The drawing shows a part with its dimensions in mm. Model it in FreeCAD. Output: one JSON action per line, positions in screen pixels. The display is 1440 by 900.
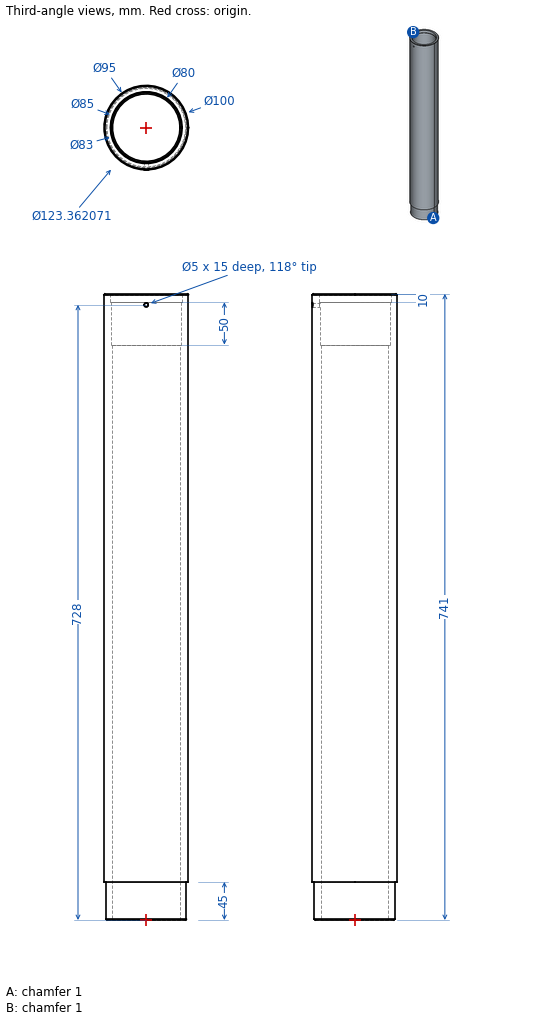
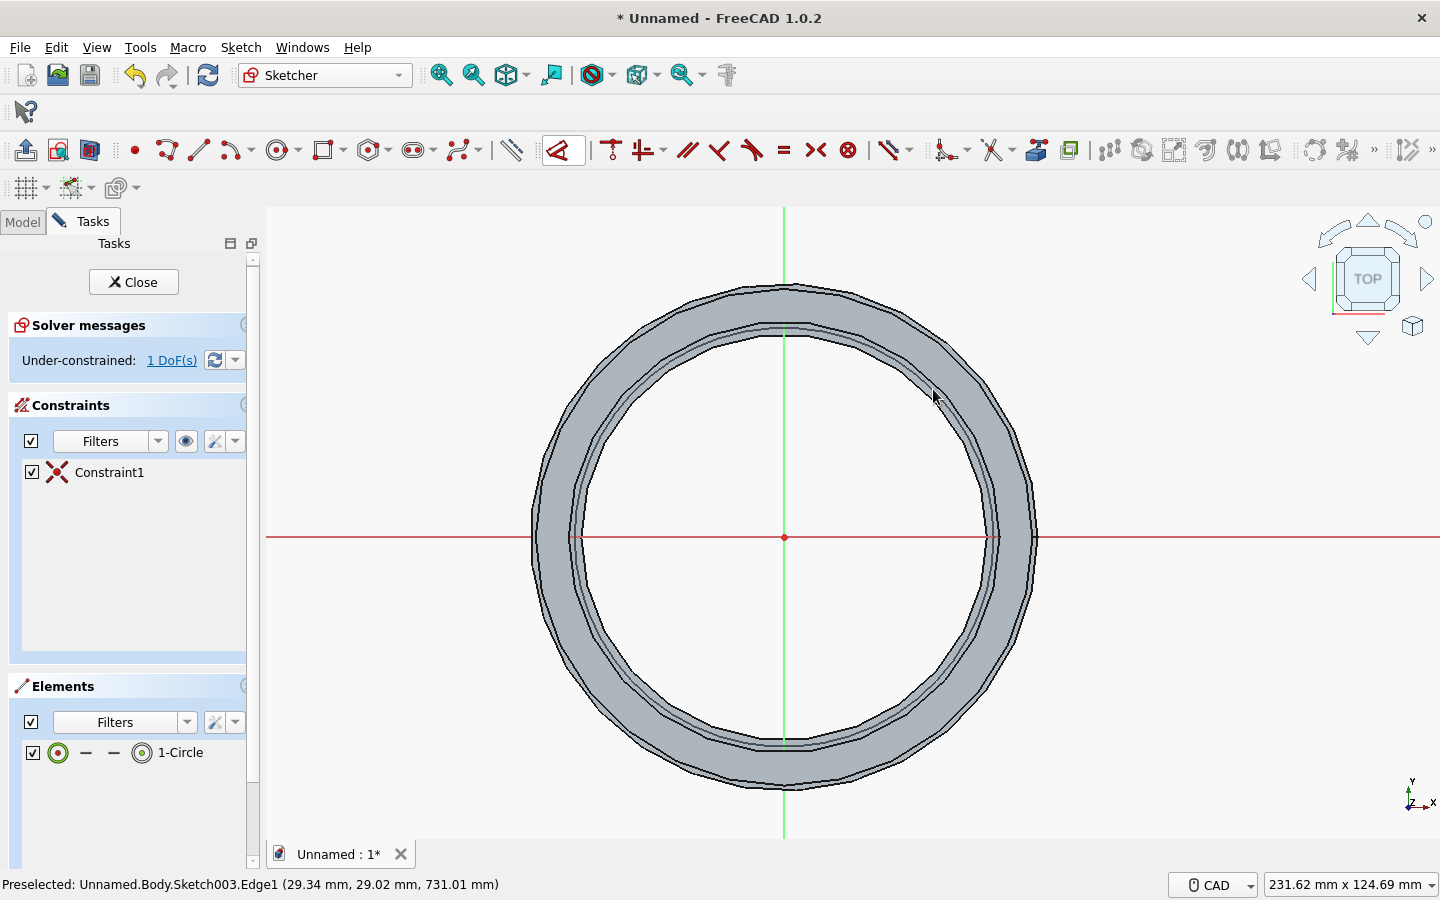
{"action": "left_click", "coordinate": [932, 389]}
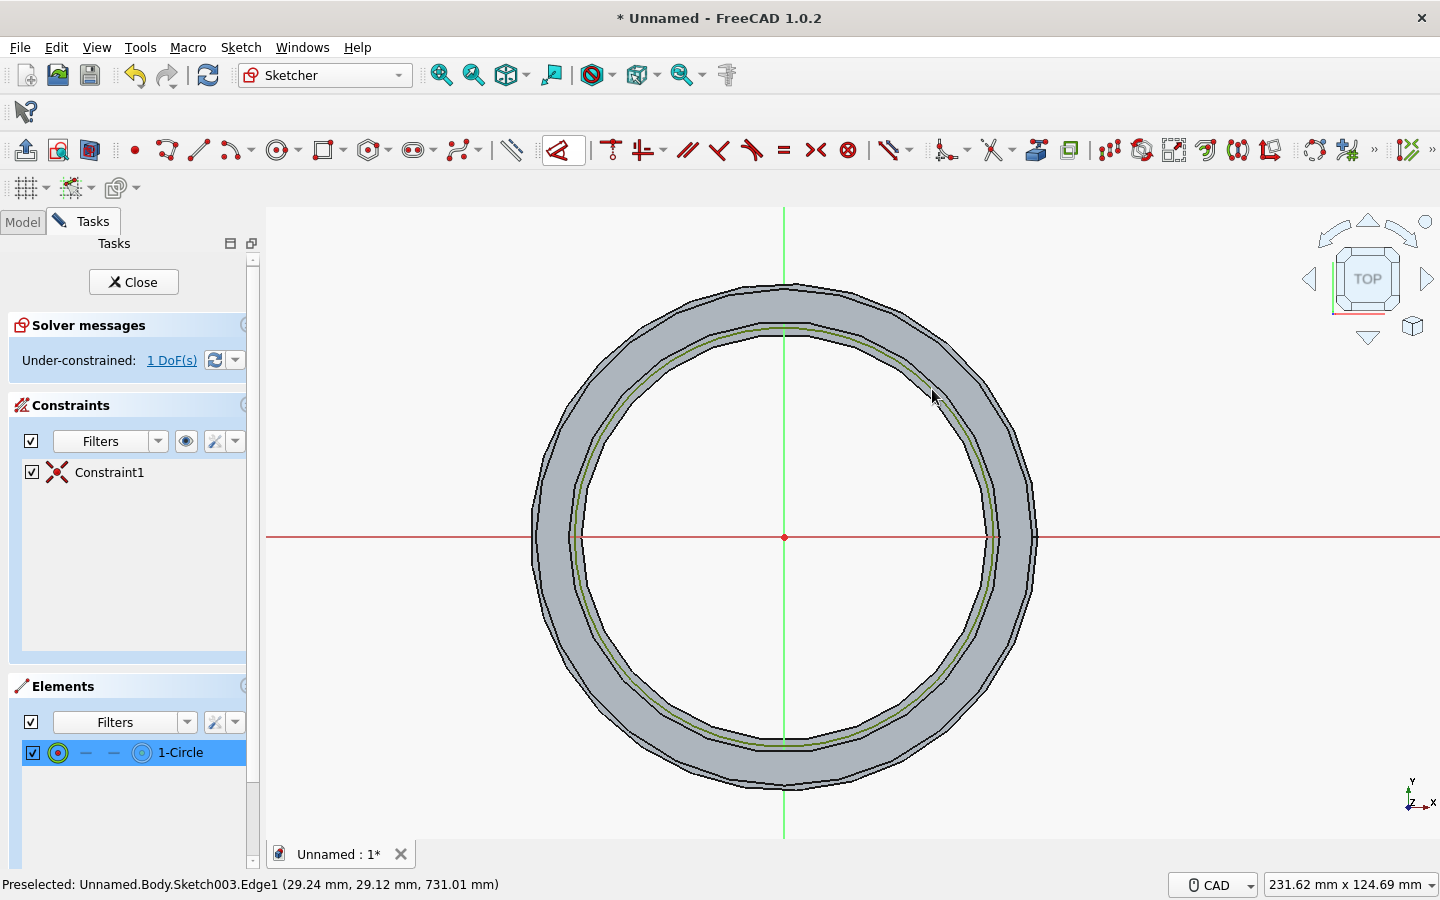
{"action": "left_click", "coordinate": [580, 150]}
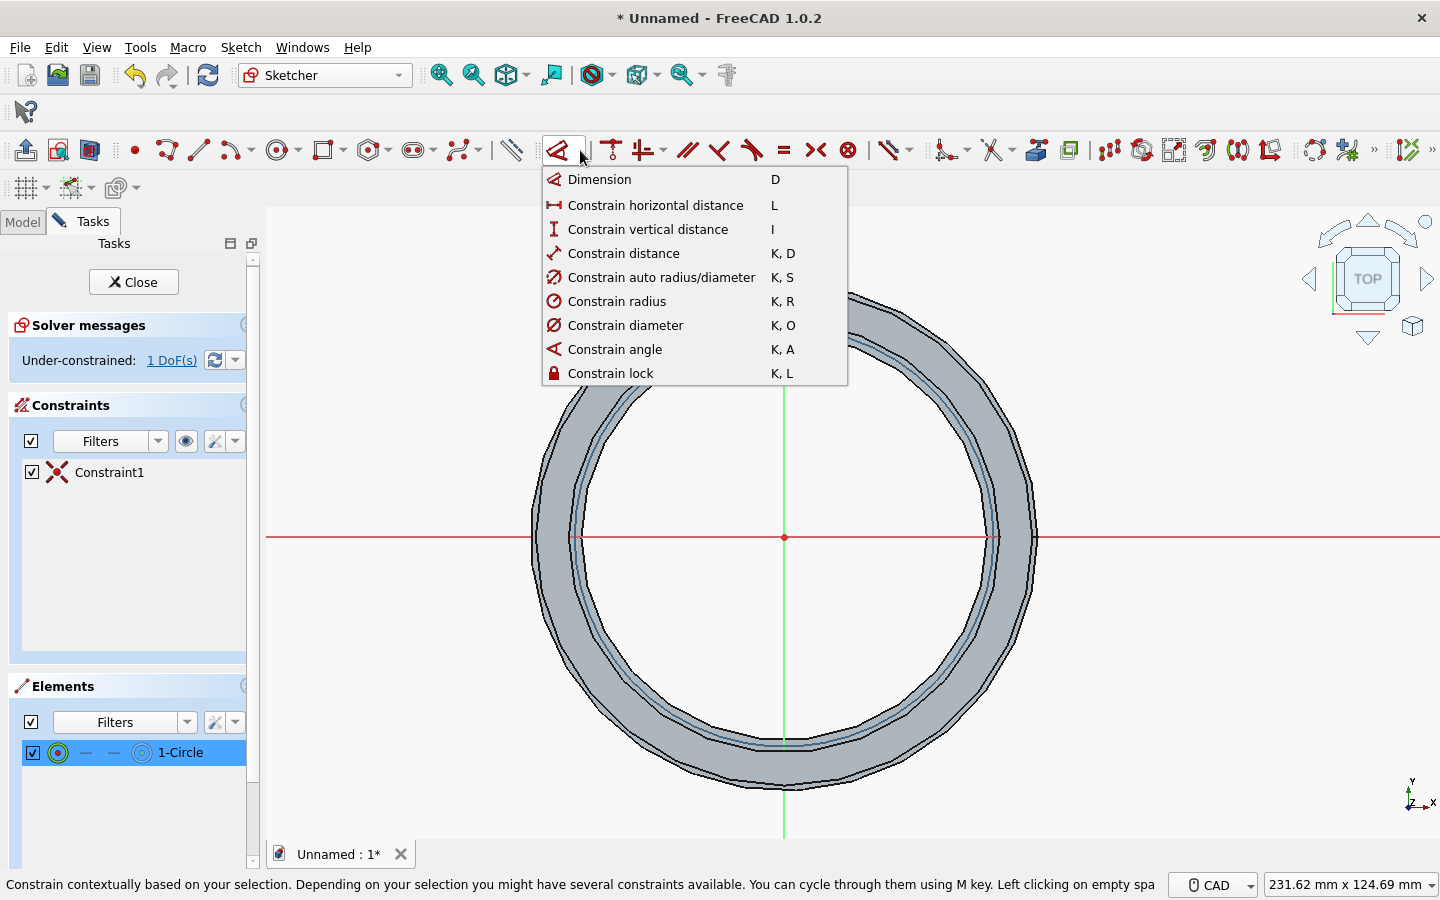
{"action": "left_click", "coordinate": [695, 325]}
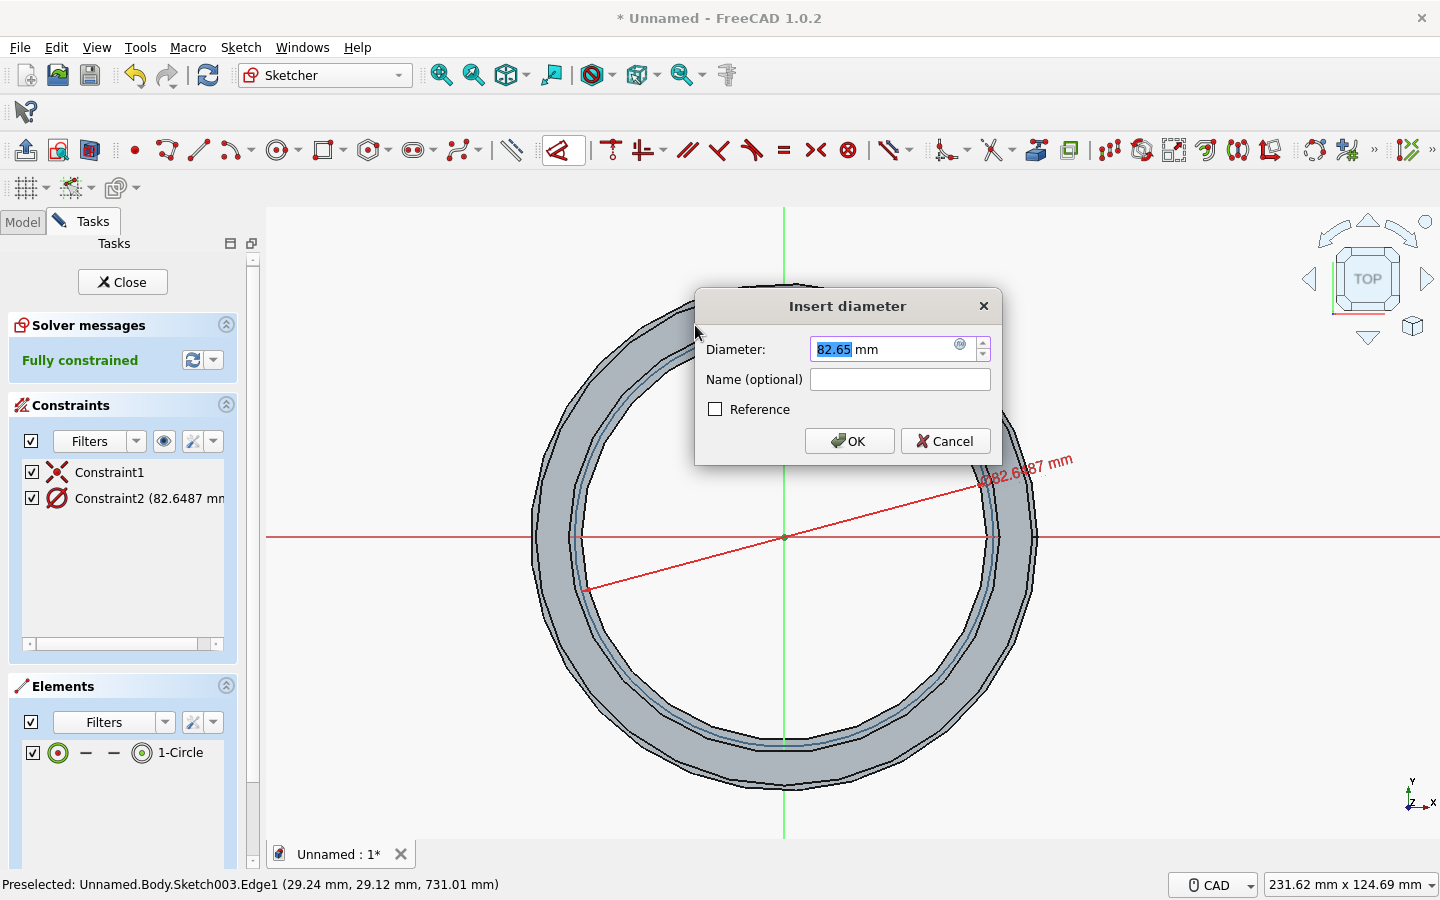
{"action": "type", "text": "83"}
{"action": "key", "text": "Return"}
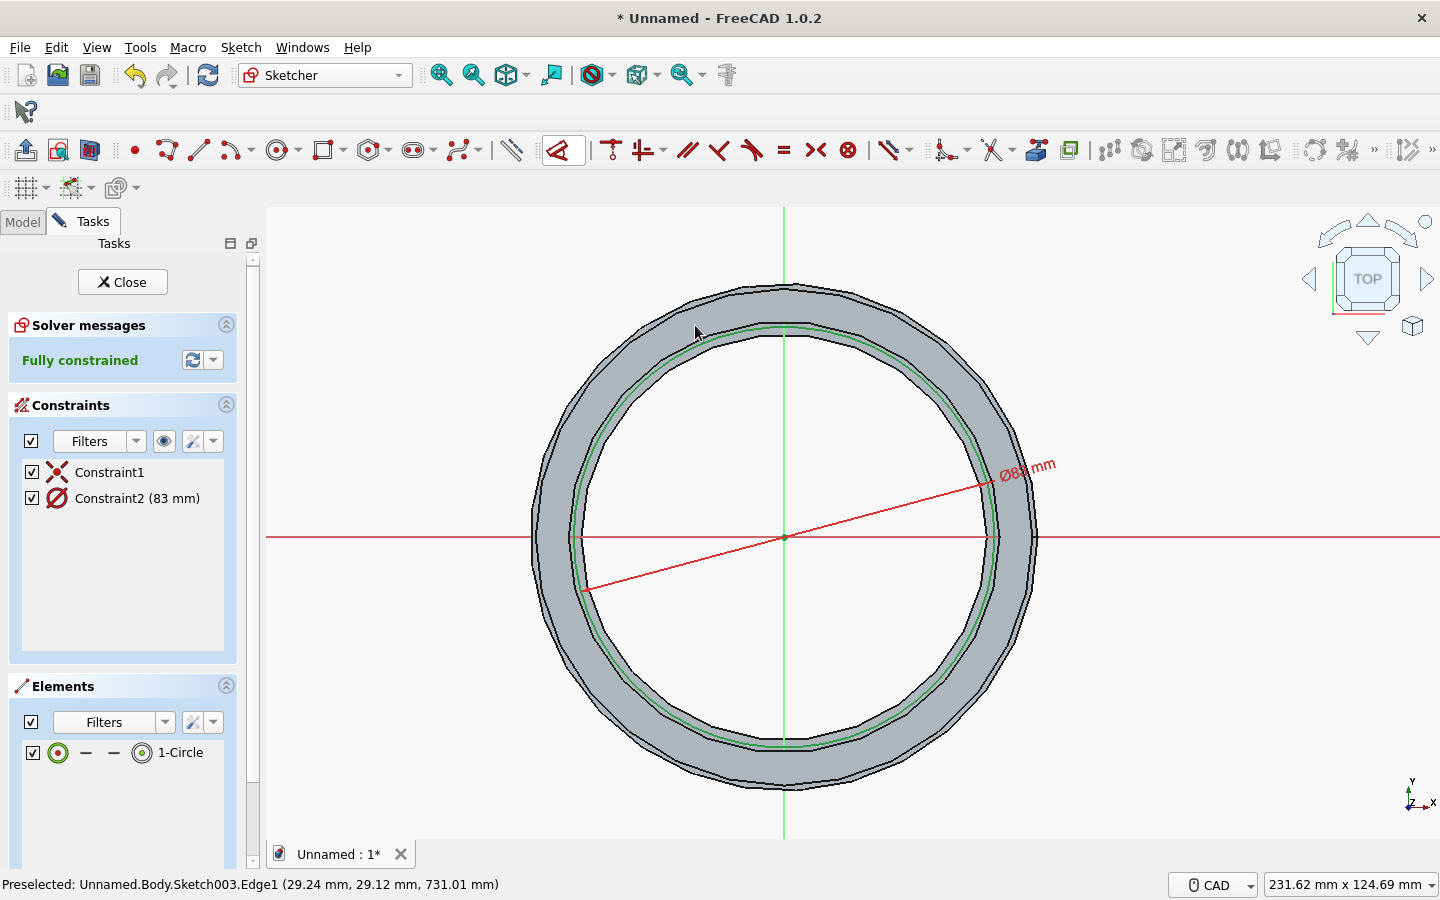
{"action": "left_click", "coordinate": [123, 282]}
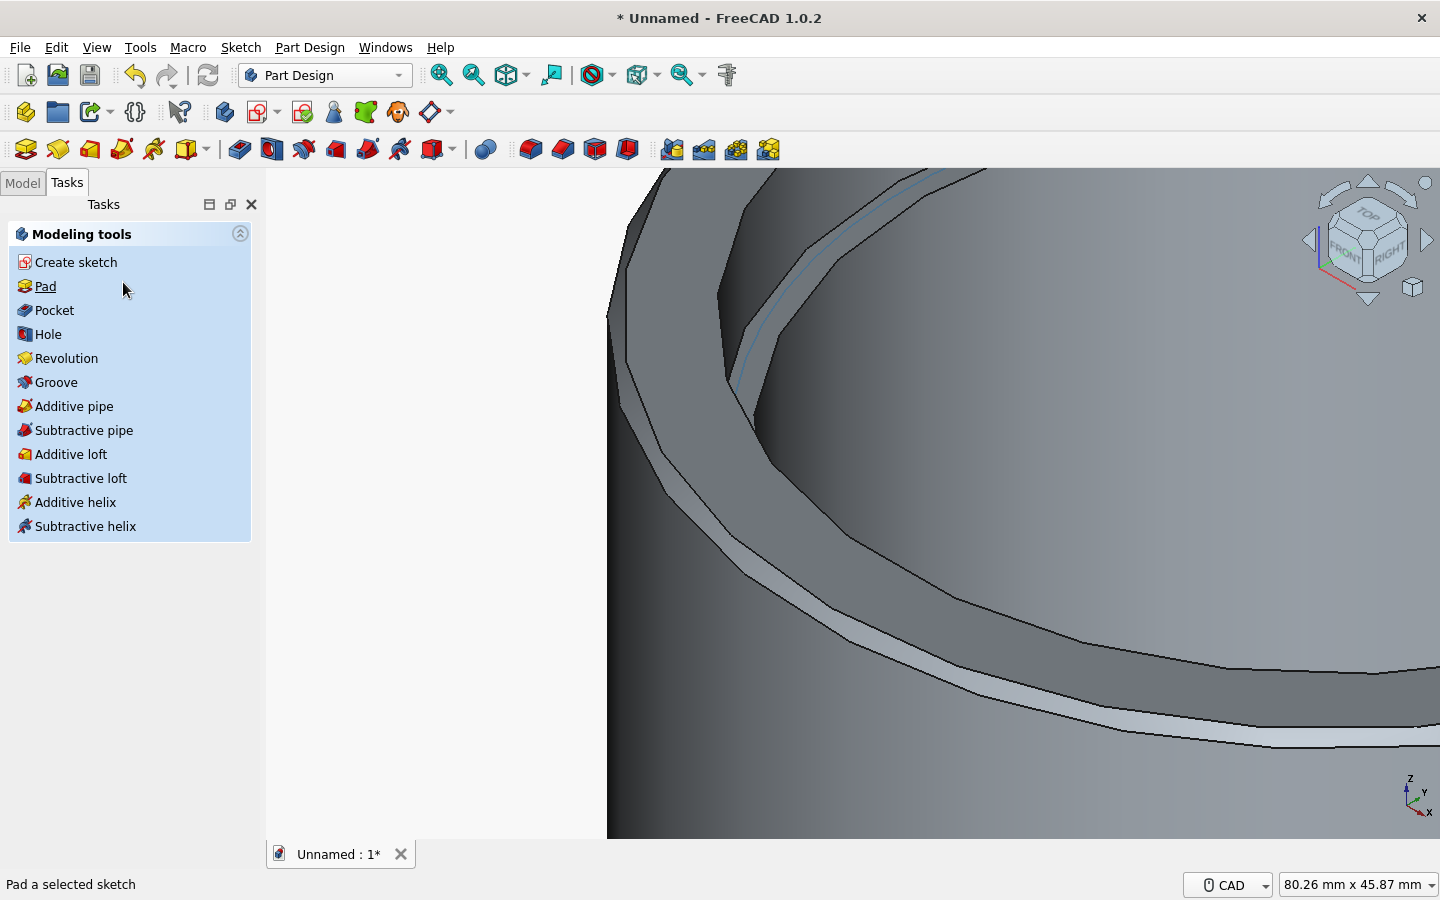
{"action": "left_click", "coordinate": [240, 150]}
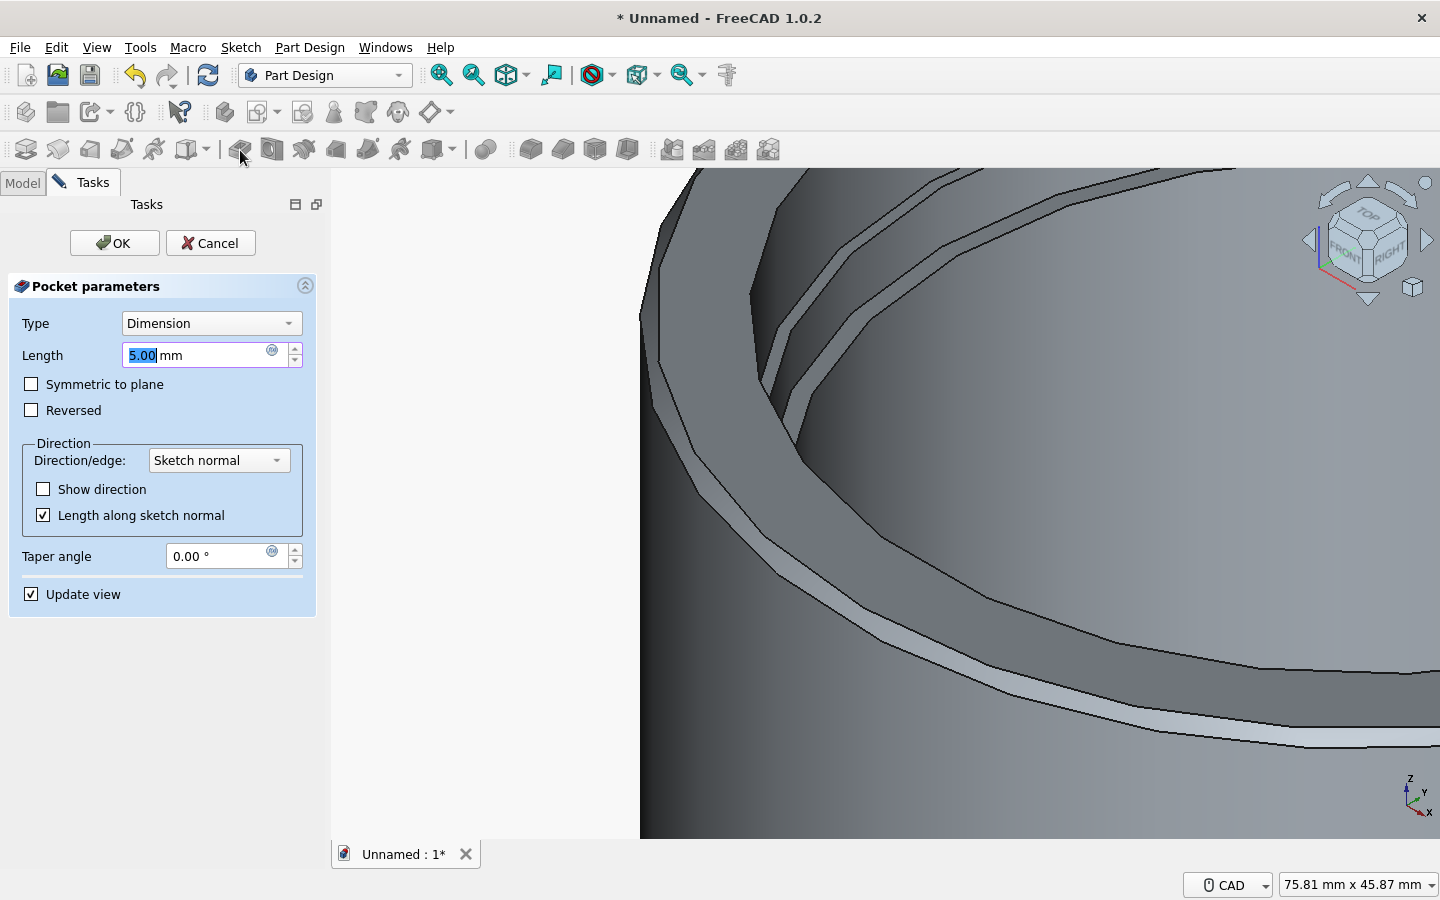
{"action": "type", "text": "50"}
{"action": "key", "text": "Tab"}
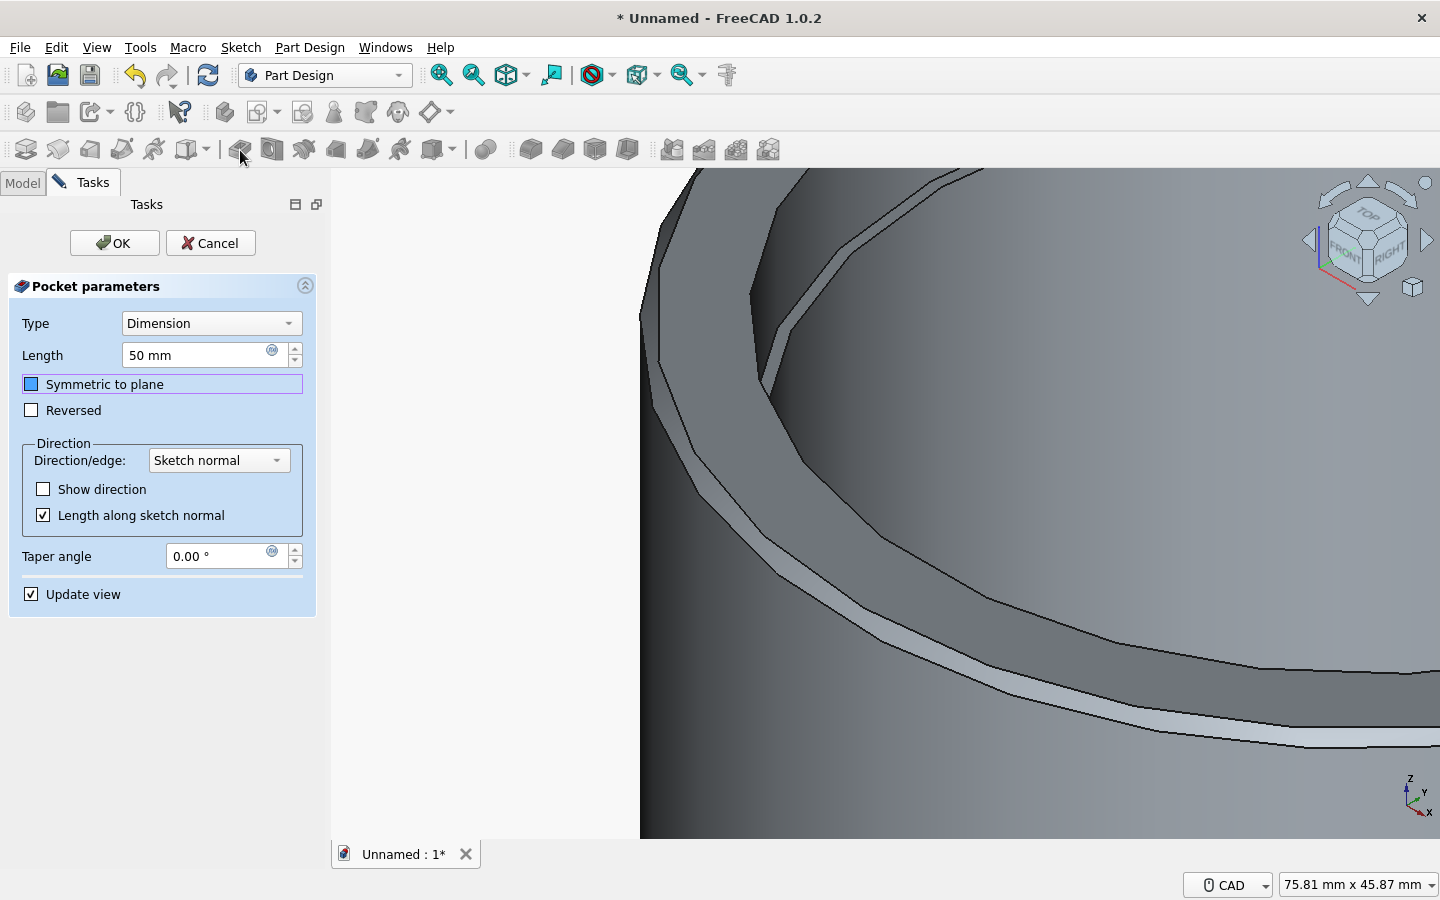
{"action": "left_click", "coordinate": [115, 243]}